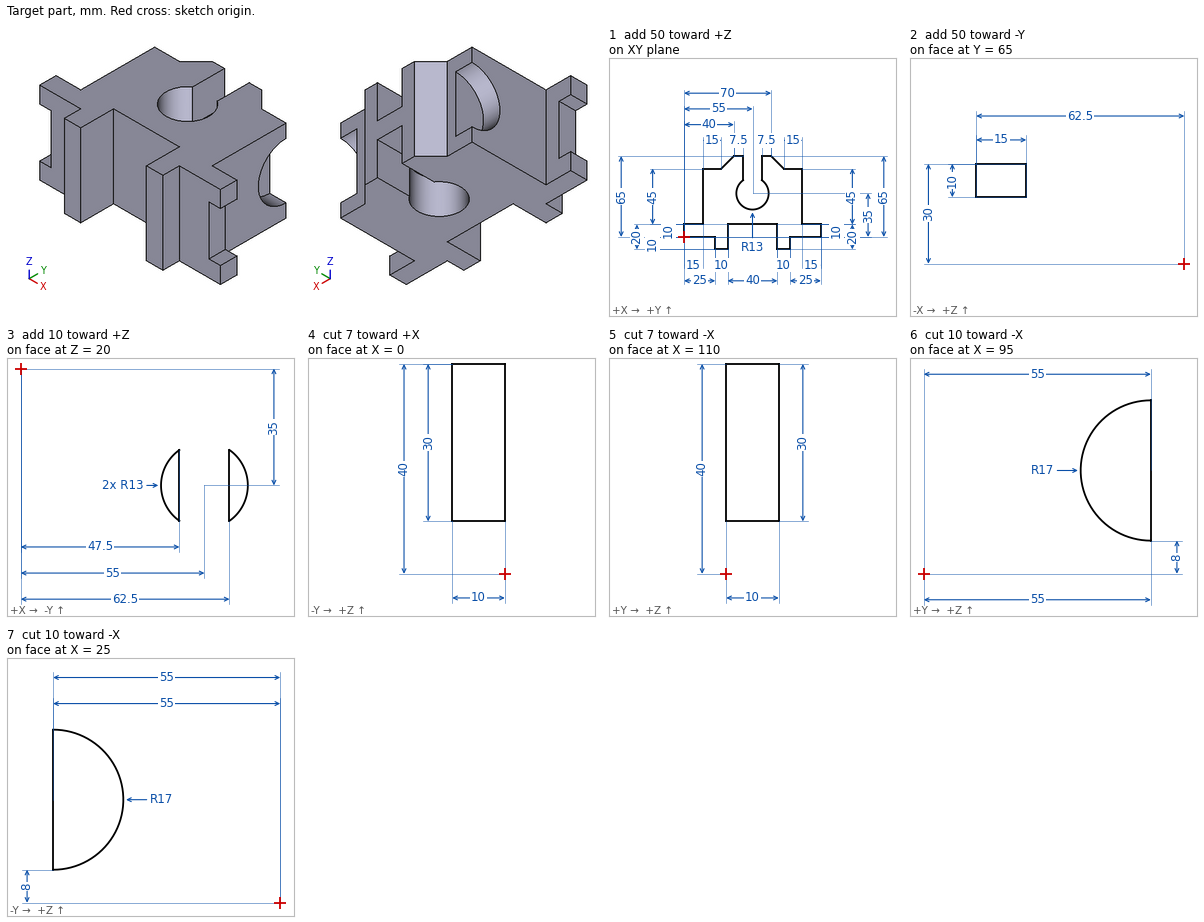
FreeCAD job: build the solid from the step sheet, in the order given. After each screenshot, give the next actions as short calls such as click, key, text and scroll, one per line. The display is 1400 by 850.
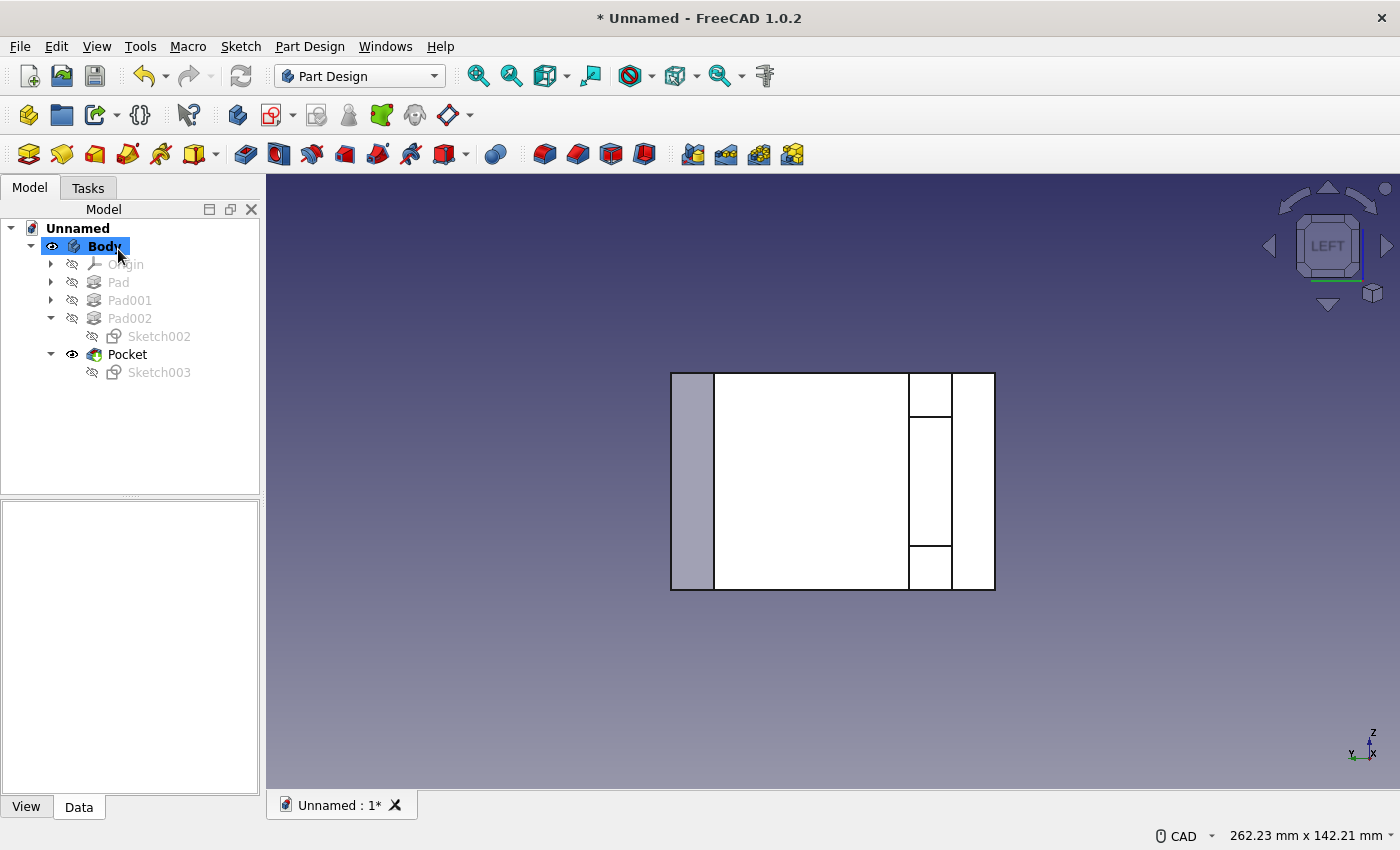
click(479, 76)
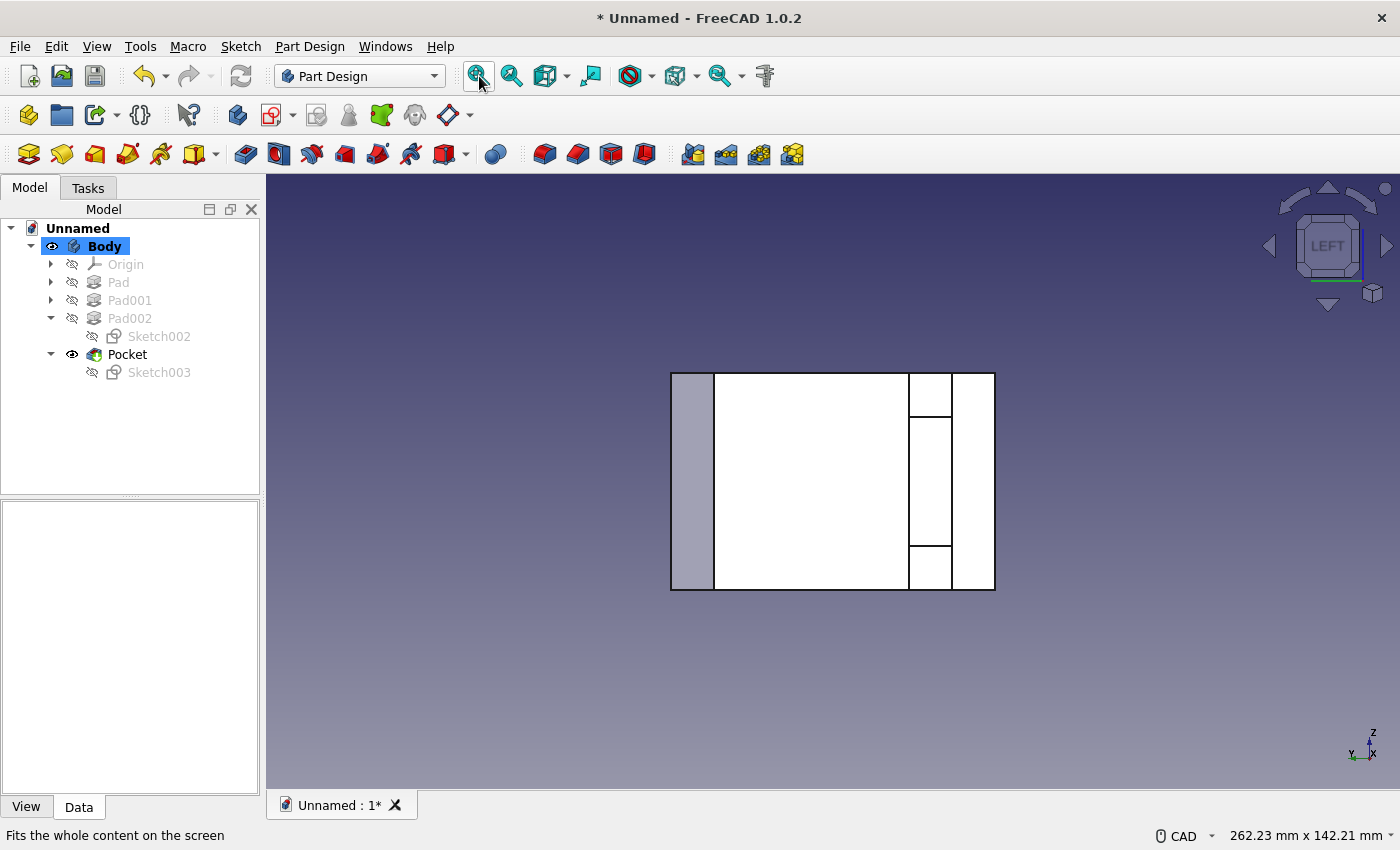
key(0)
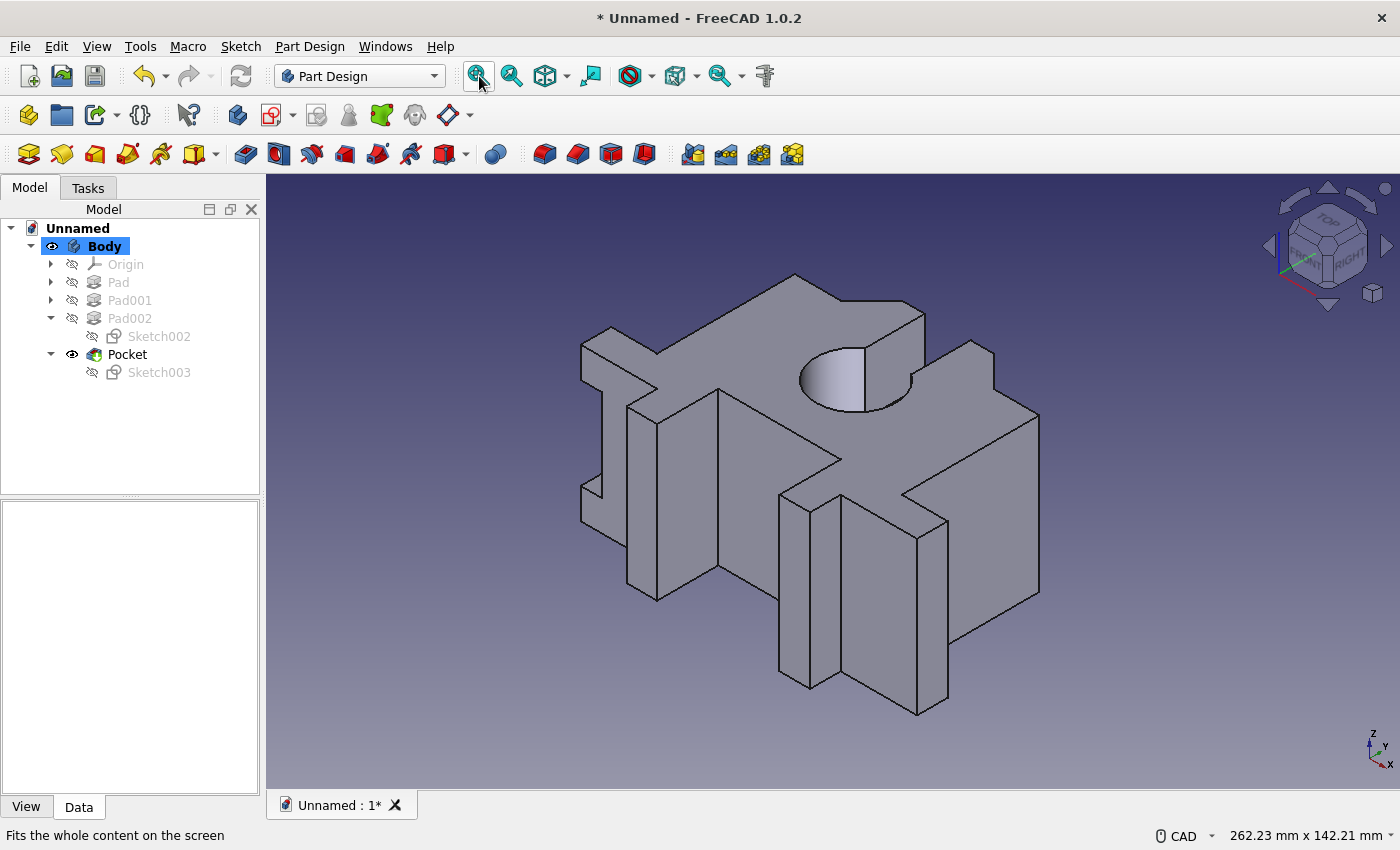
click(932, 567)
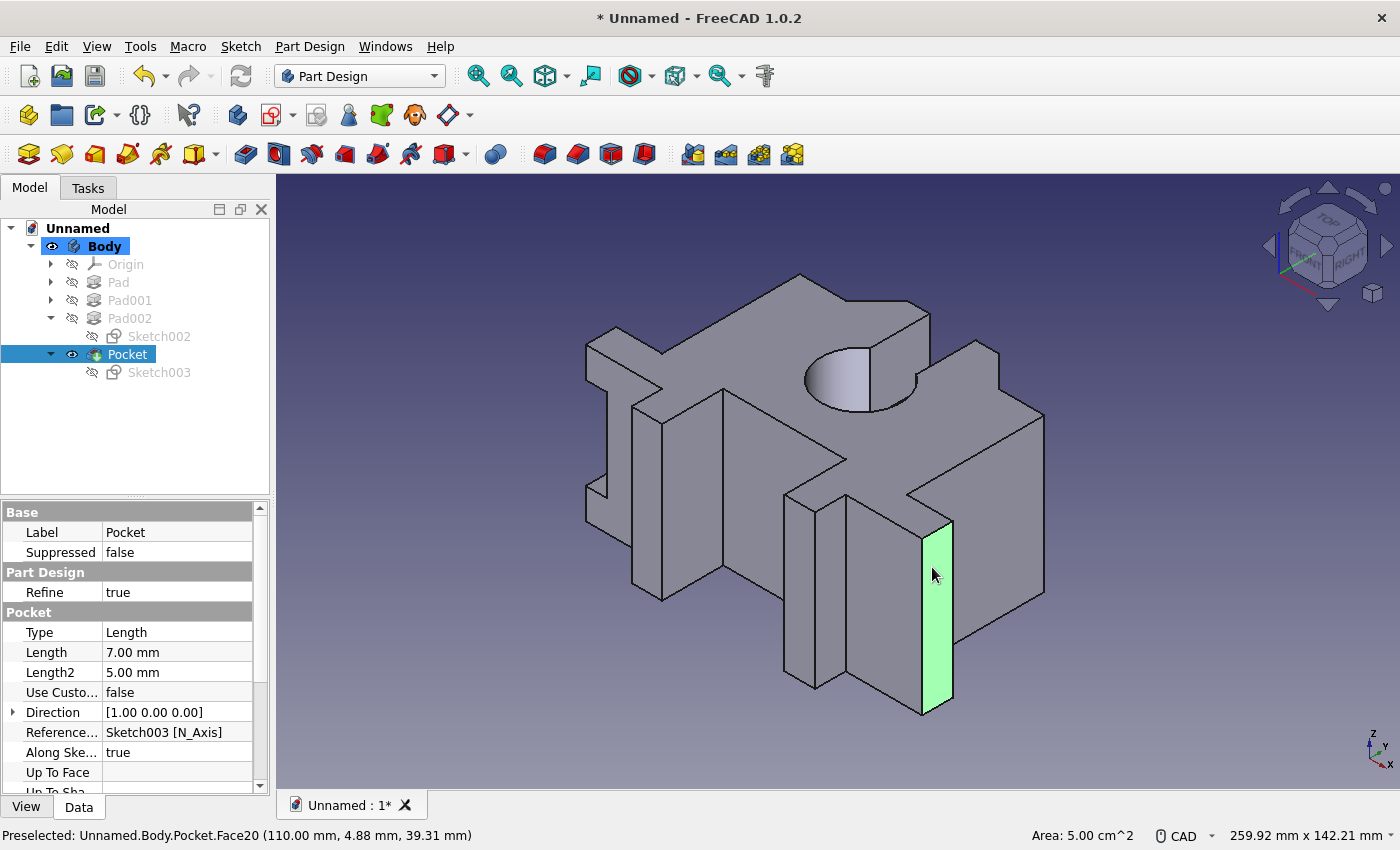
click(270, 116)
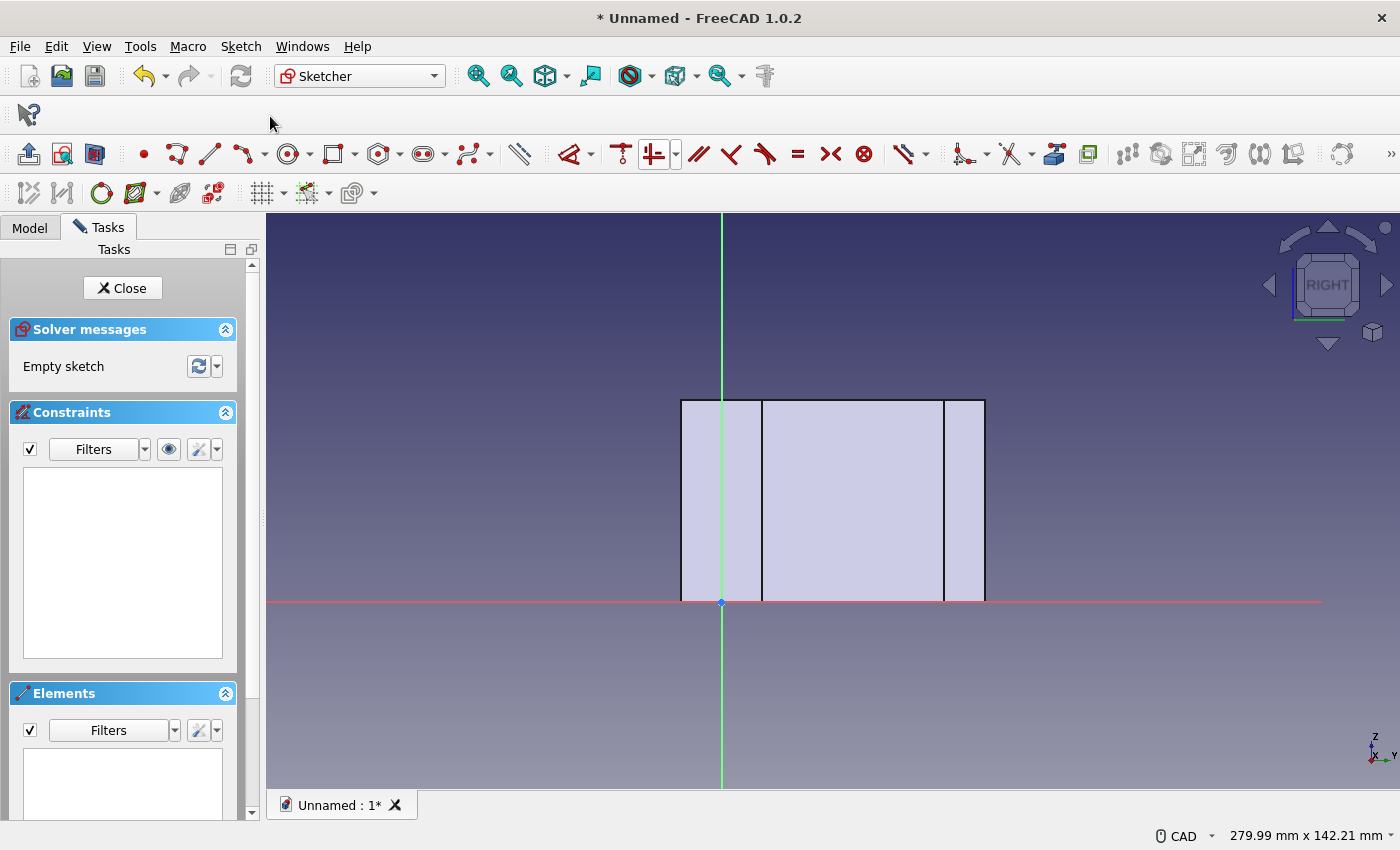
scroll(723, 538, up, 4)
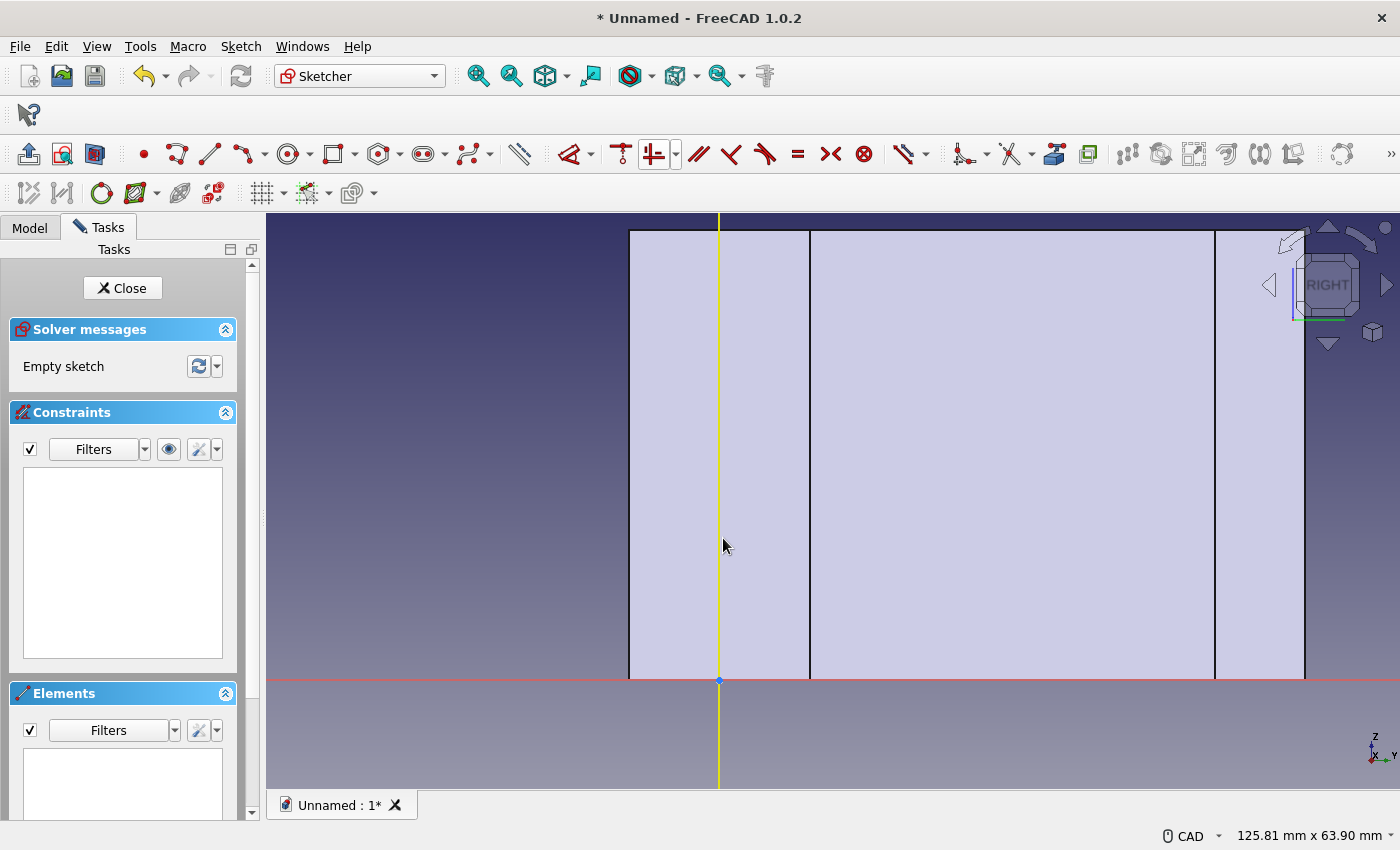
click(332, 154)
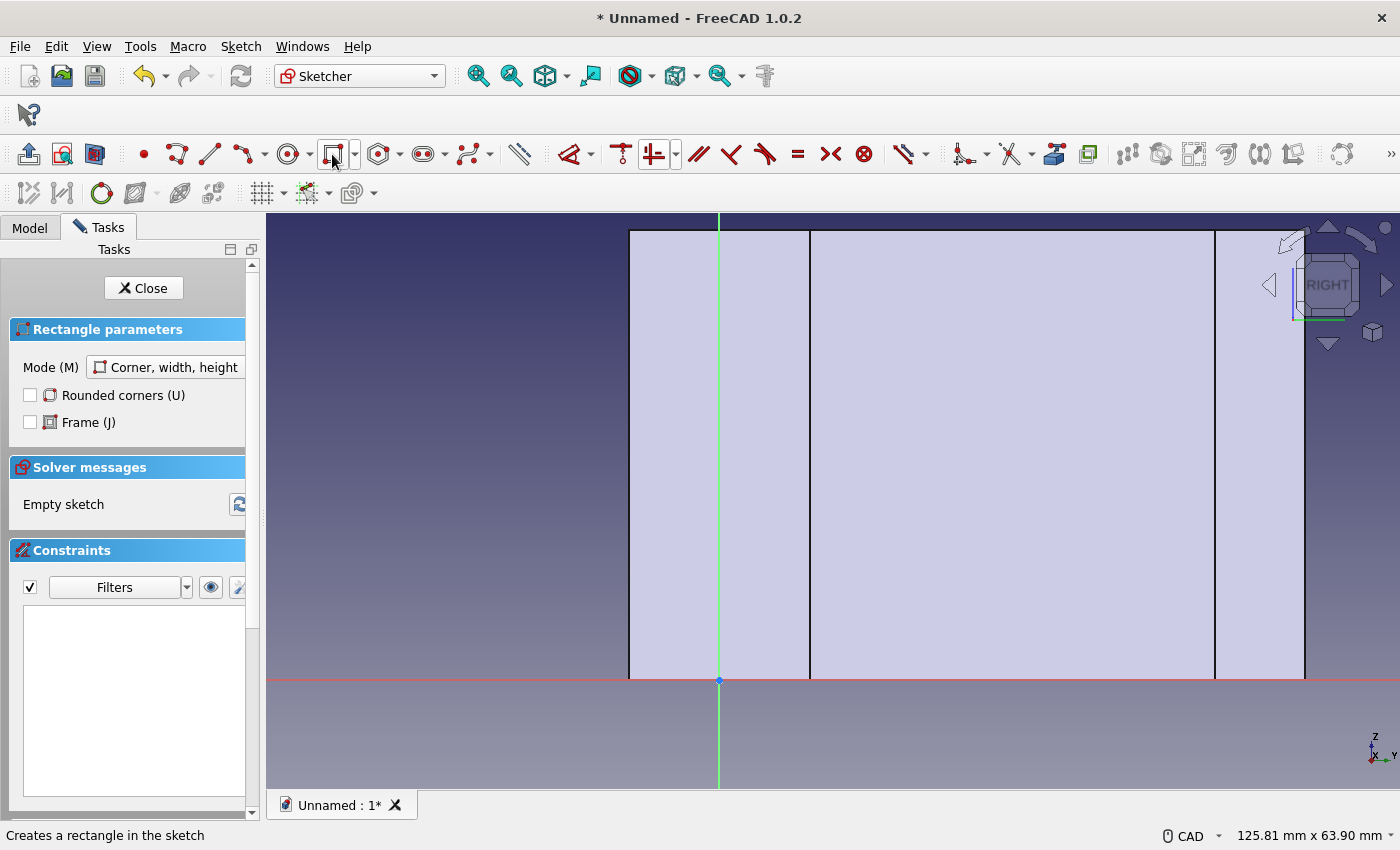
click(719, 320)
move(810, 590)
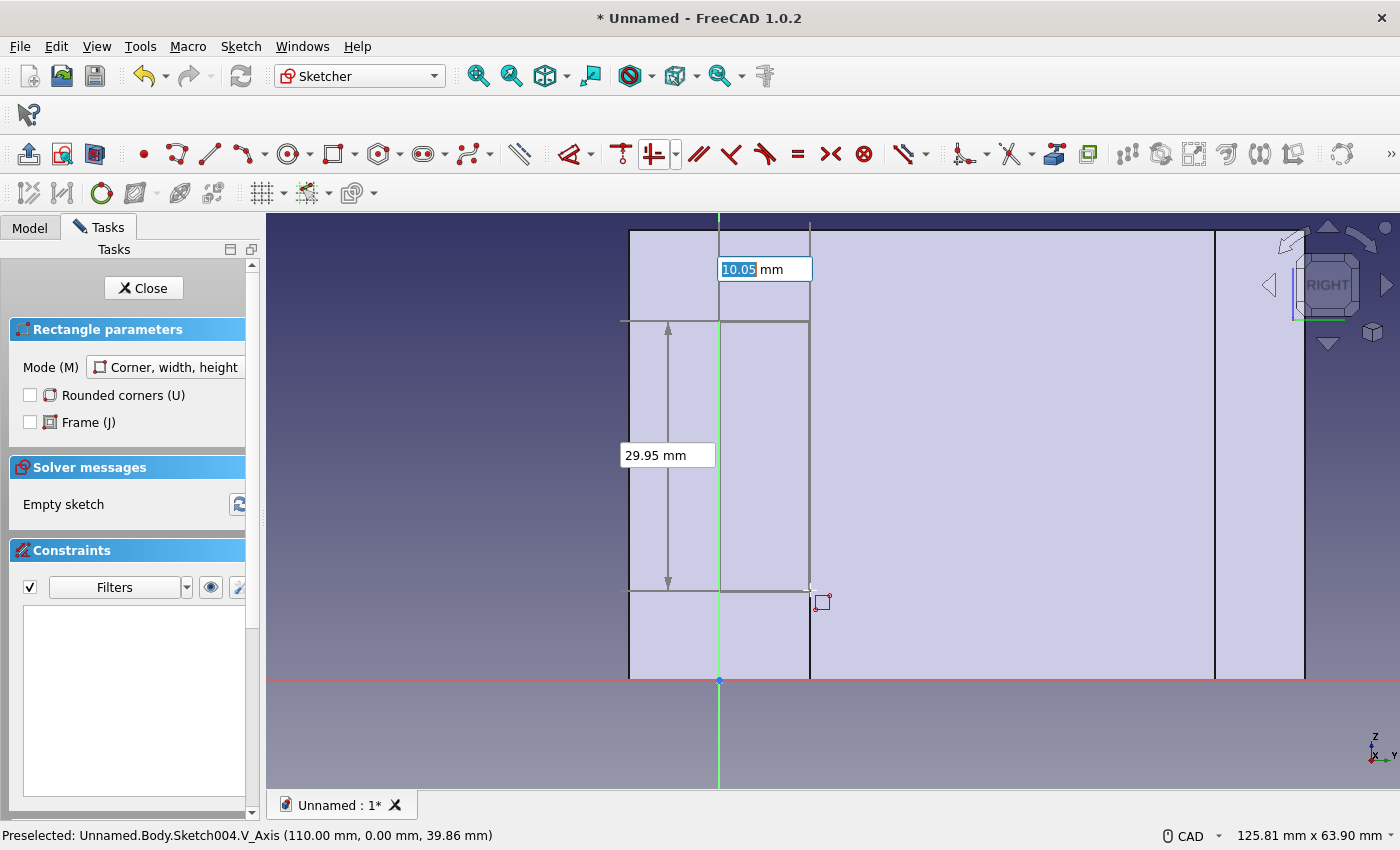
text(10)
key(Tab)
text(30)
key(Return)
key(Escape)